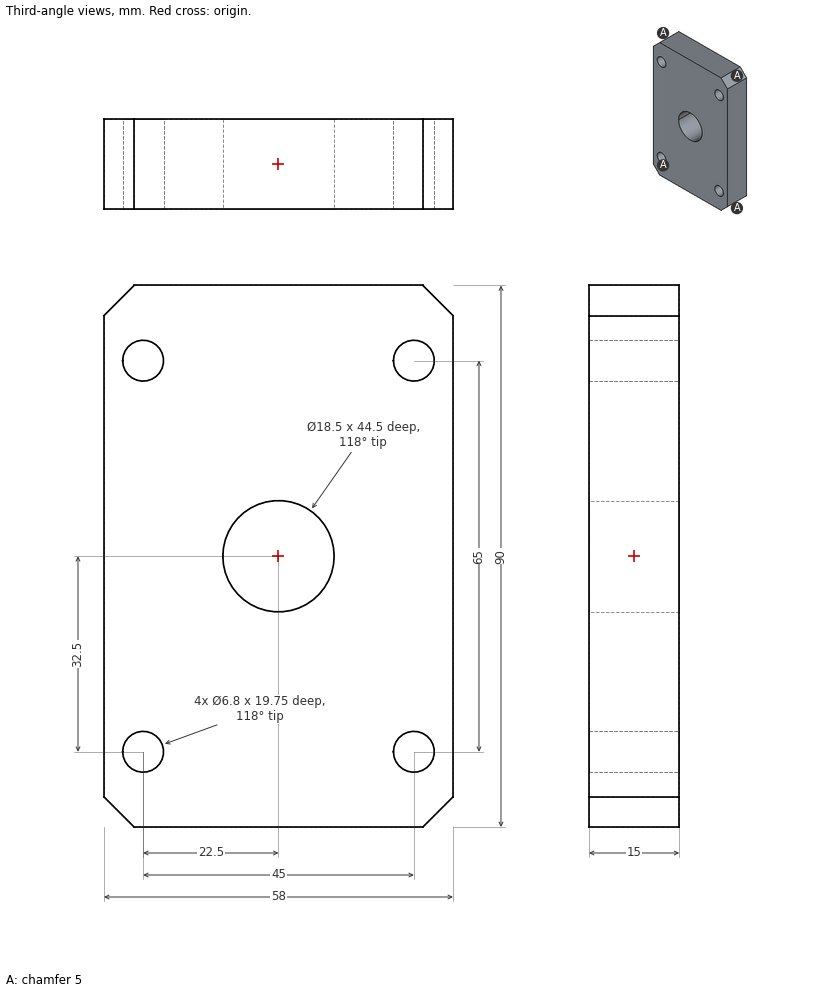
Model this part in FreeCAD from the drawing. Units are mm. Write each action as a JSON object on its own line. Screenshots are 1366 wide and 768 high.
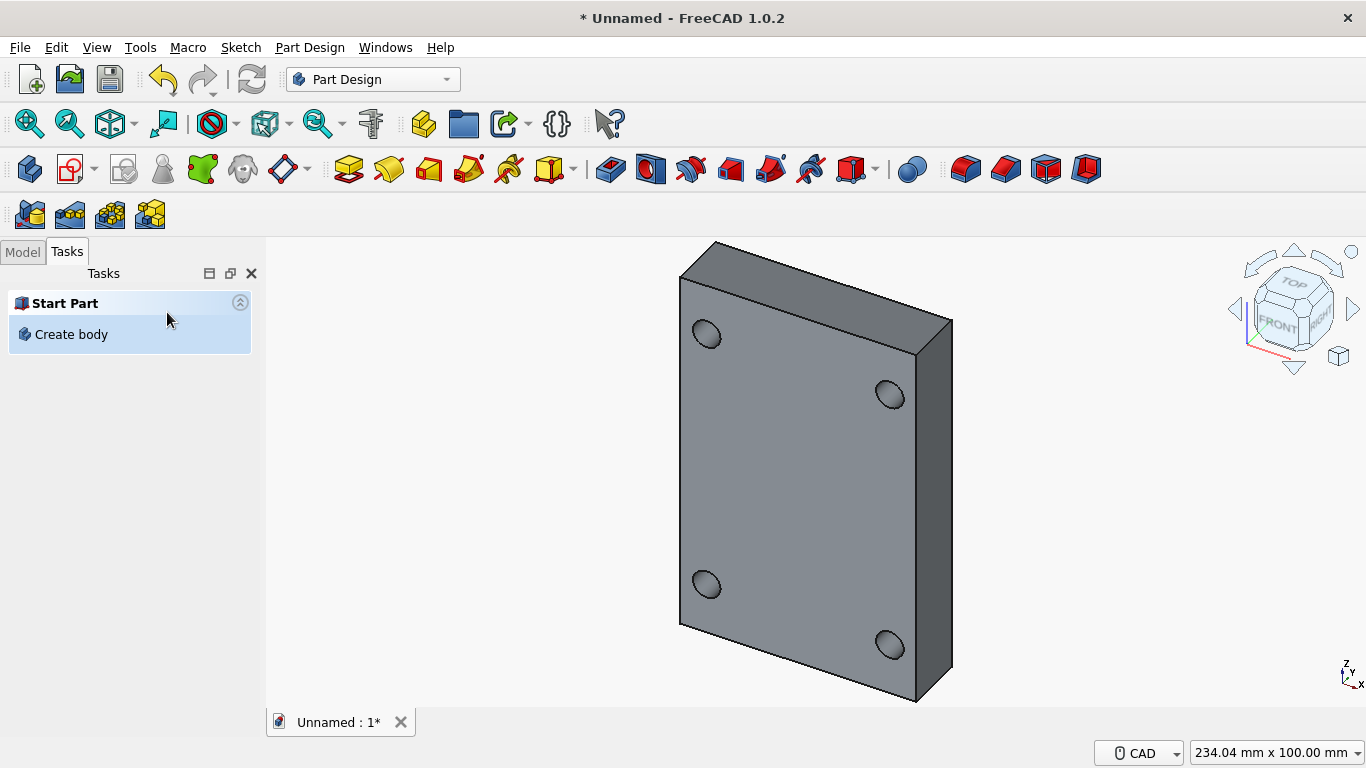
{"action": "key", "text": "4"}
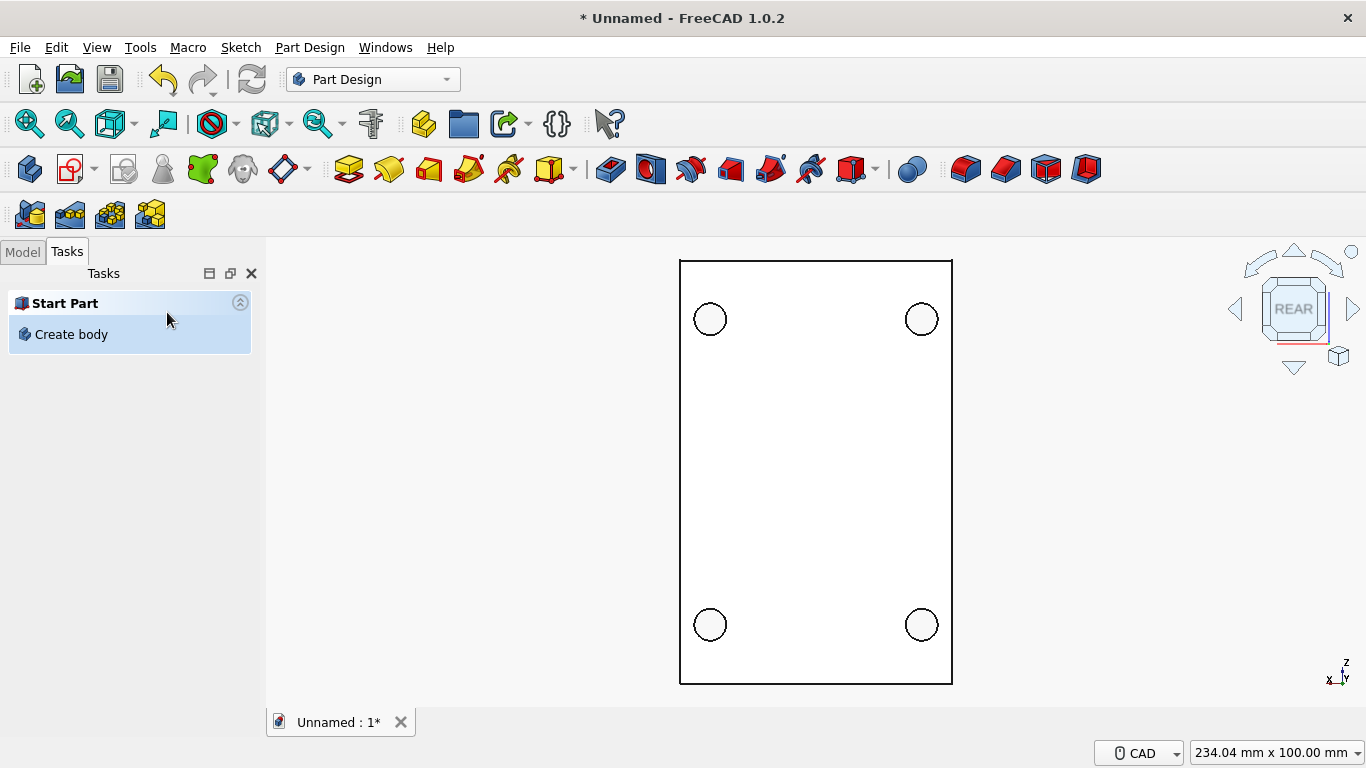
{"action": "left_click", "coordinate": [816, 471]}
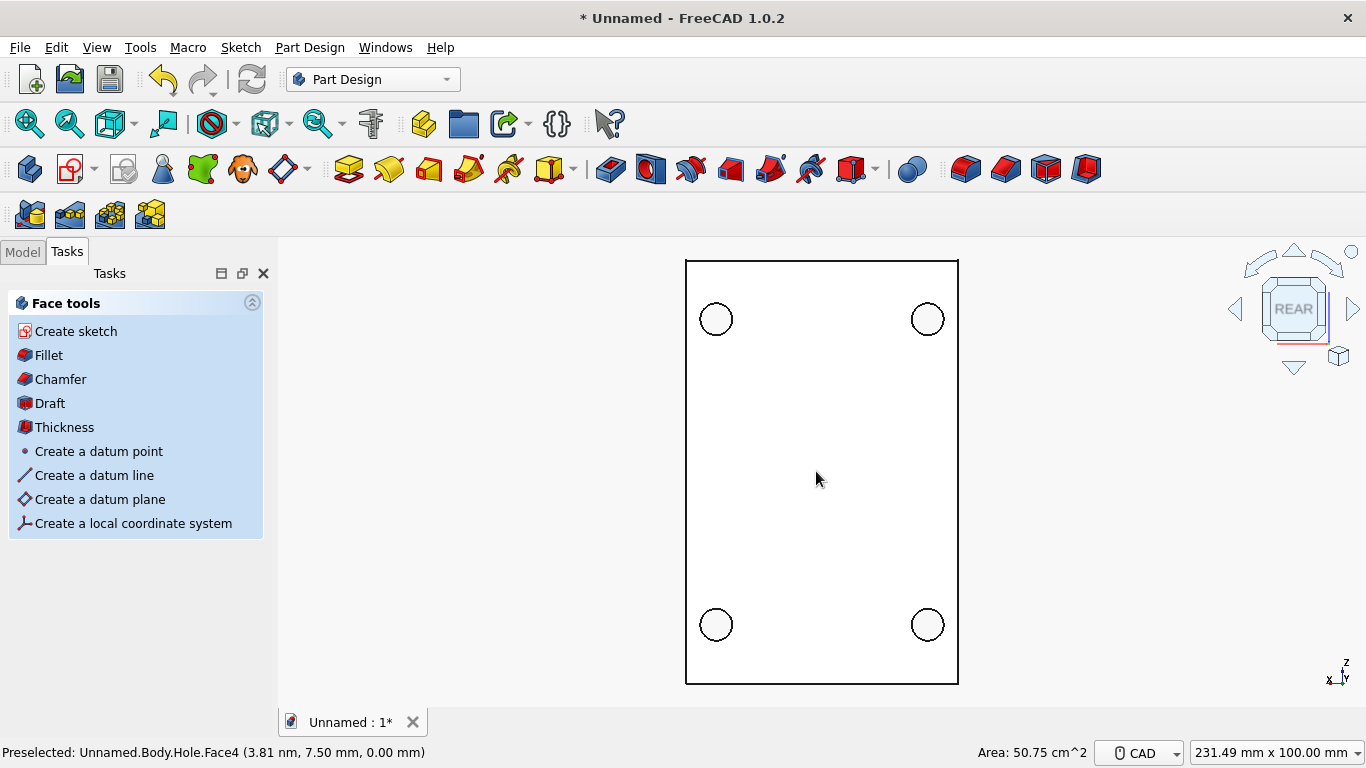
{"action": "left_click", "coordinate": [70, 170]}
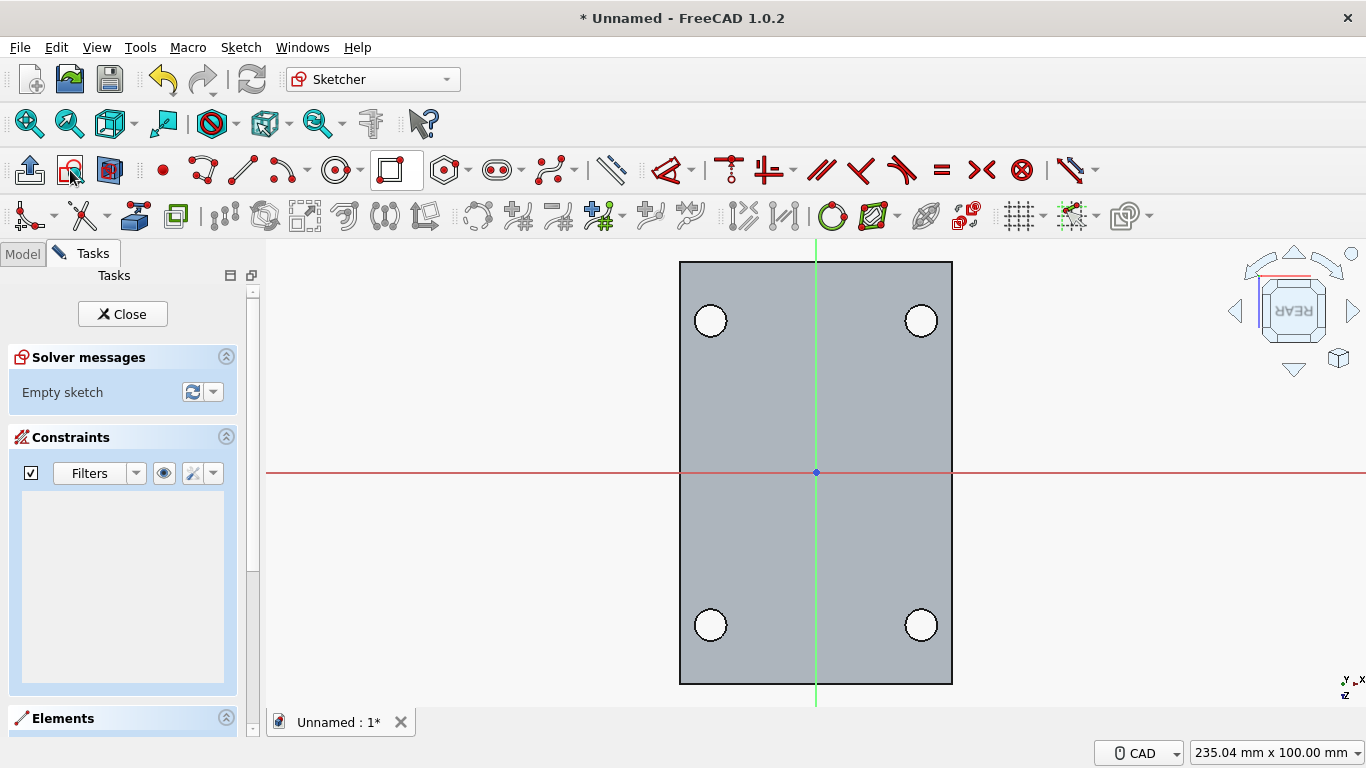
{"action": "scroll", "coordinate": [846, 473], "scroll_direction": "up", "scroll_amount": 6}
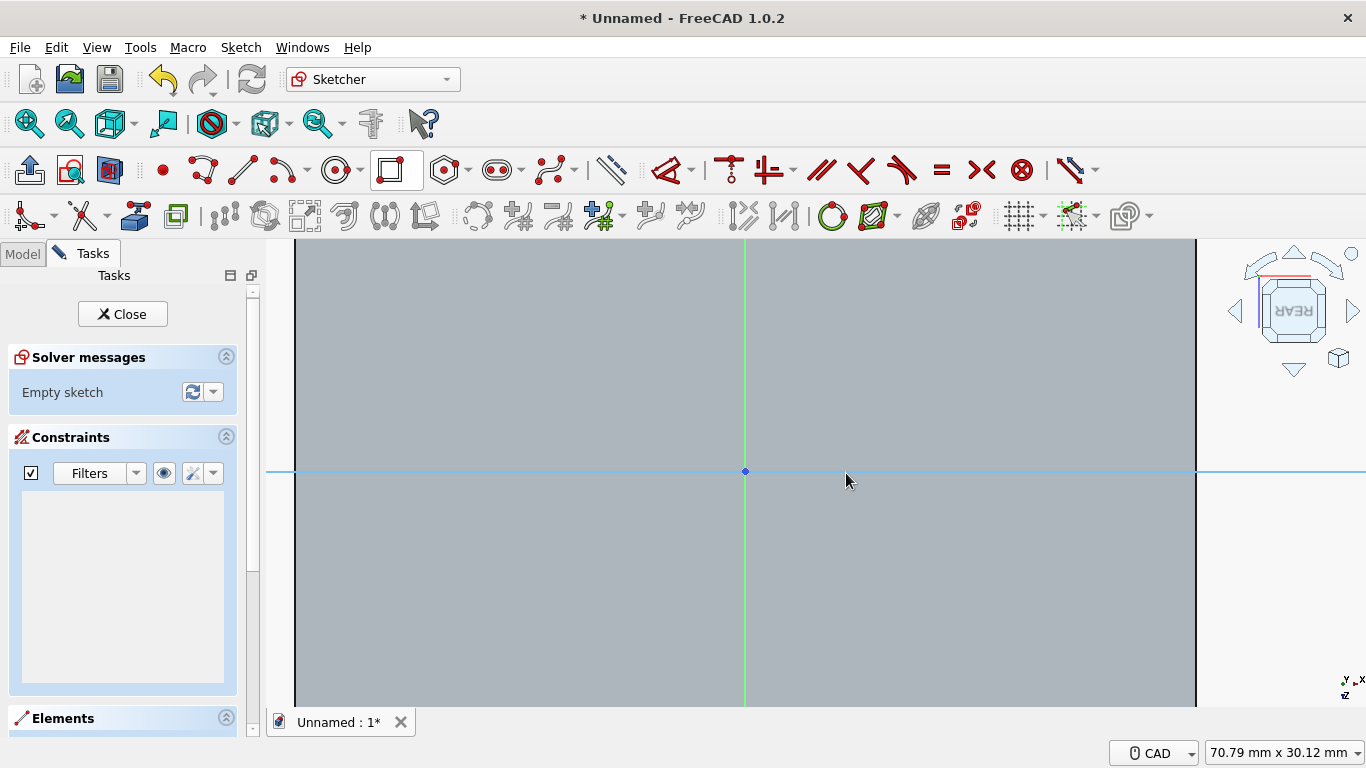
{"action": "key", "text": "g c"}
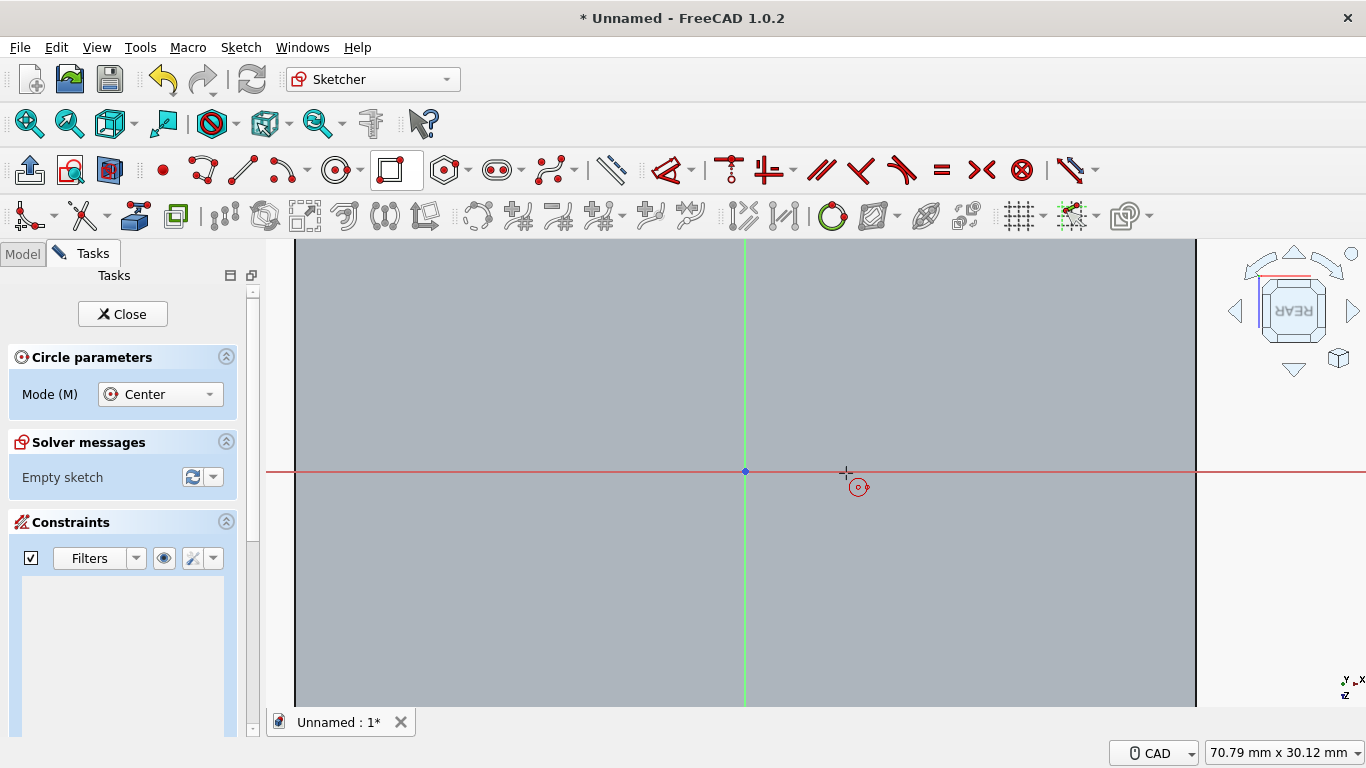
{"action": "left_click", "coordinate": [745, 472]}
{"action": "left_click", "coordinate": [847, 370]}
{"action": "key", "text": "Escape"}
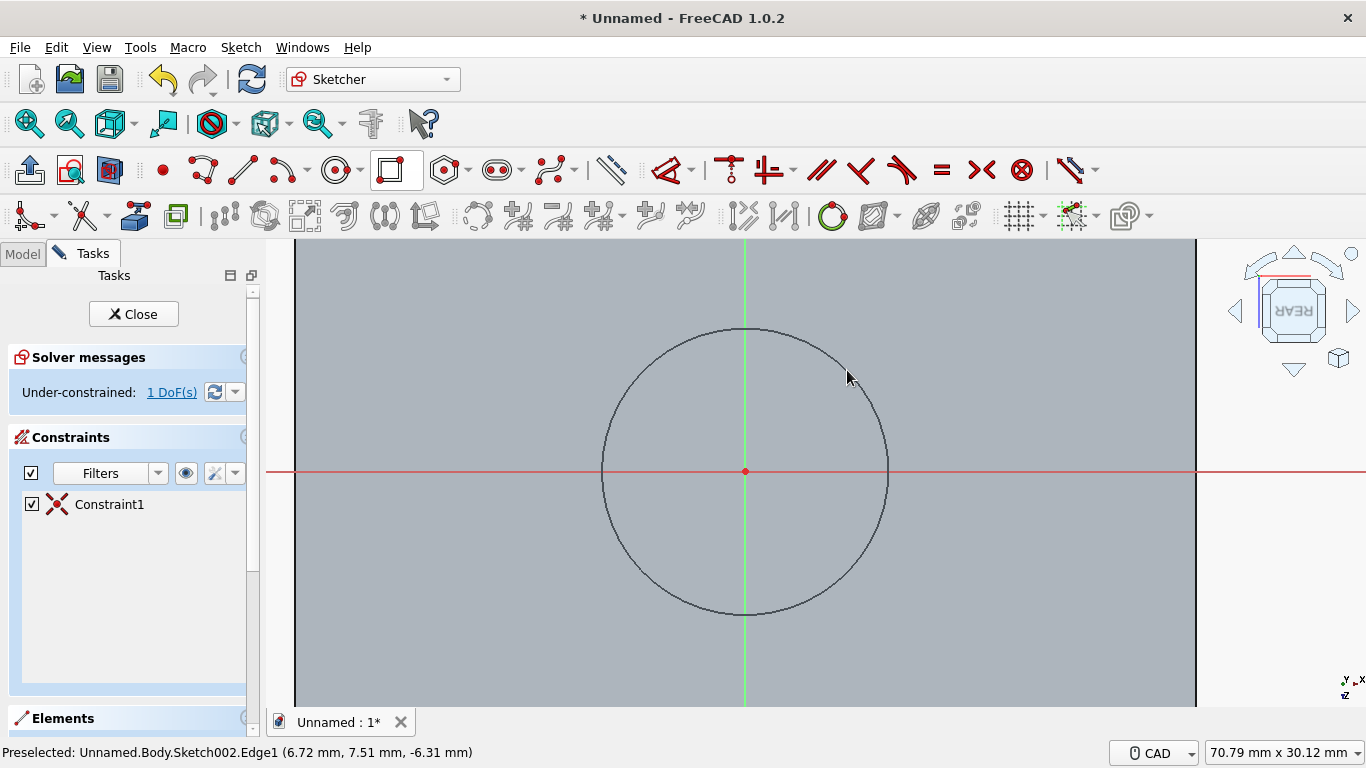
{"action": "key", "text": "d"}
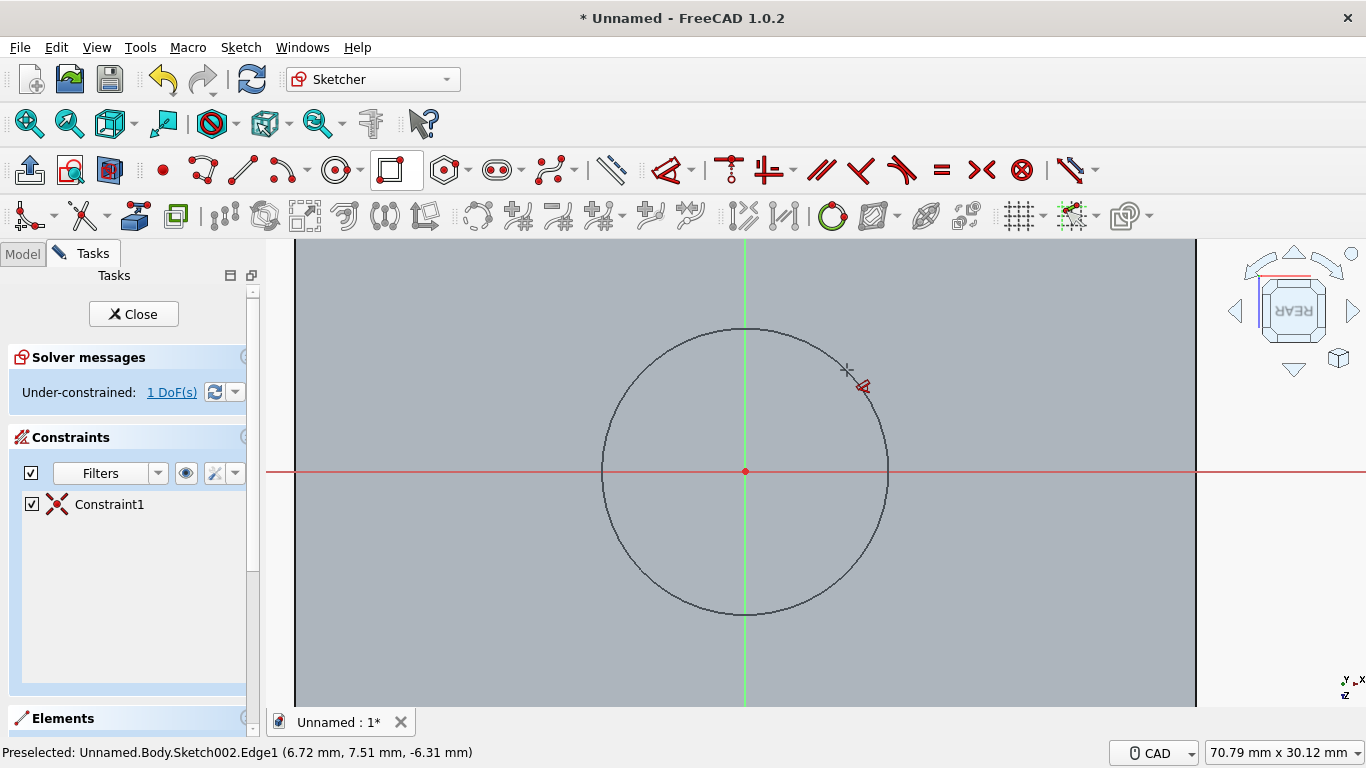
{"action": "left_click", "coordinate": [846, 370]}
{"action": "left_click", "coordinate": [869, 347]}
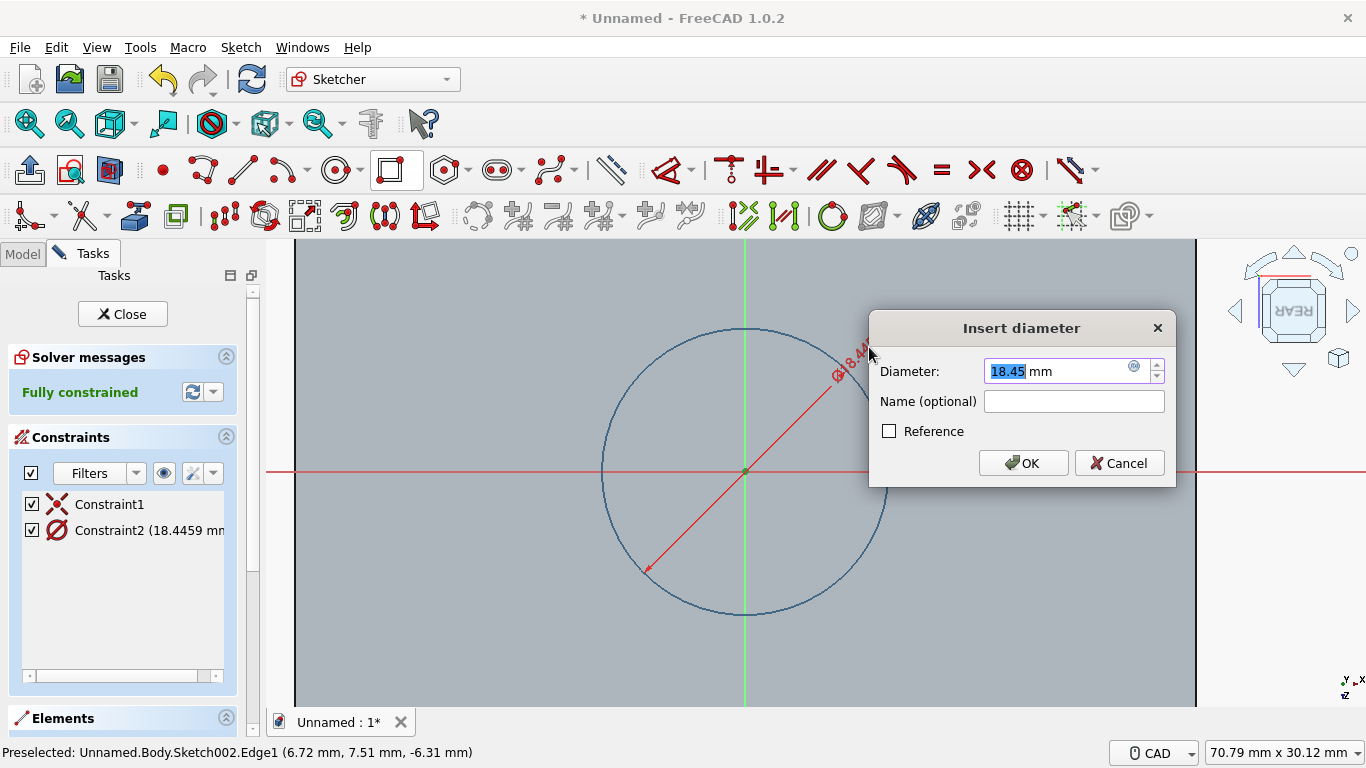
{"action": "type", "text": "18.5"}
{"action": "key", "text": "Return"}
{"action": "key", "text": "Escape"}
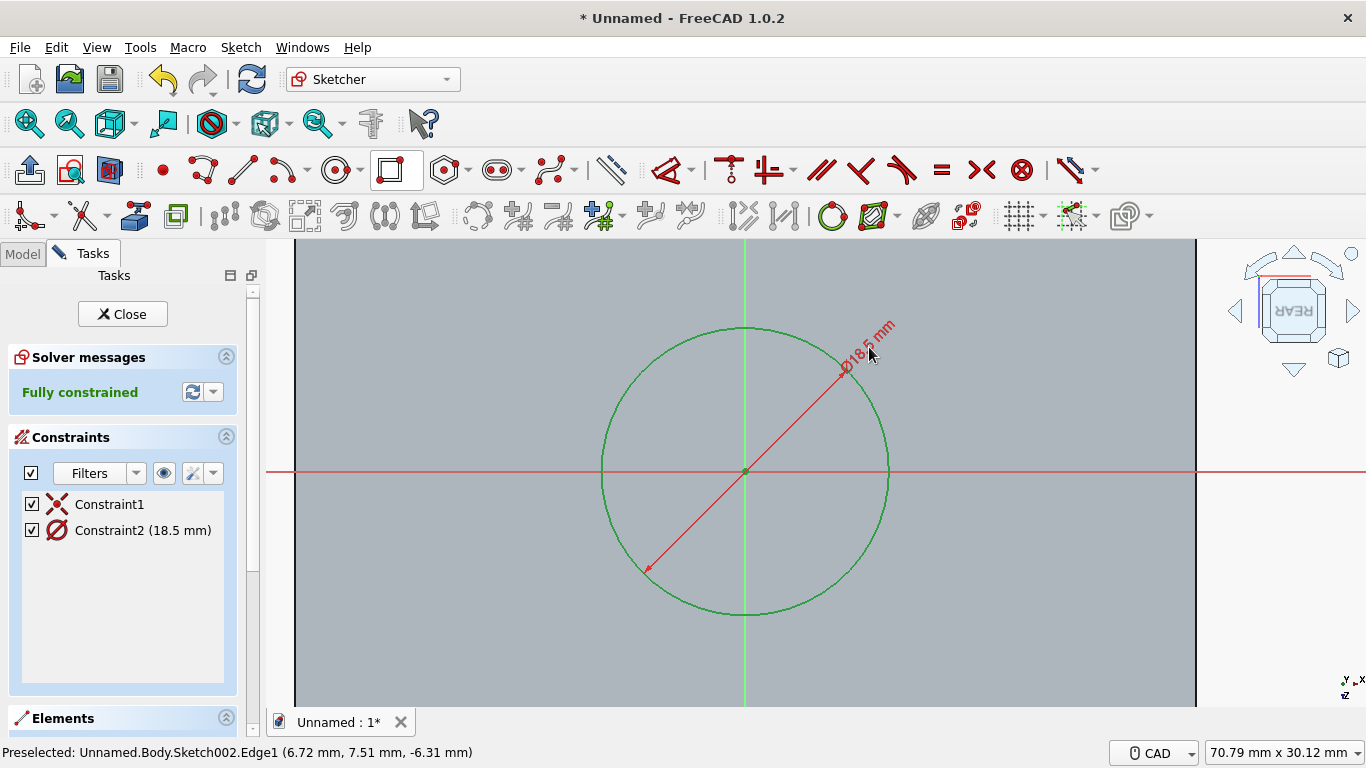
{"action": "left_click", "coordinate": [123, 314]}